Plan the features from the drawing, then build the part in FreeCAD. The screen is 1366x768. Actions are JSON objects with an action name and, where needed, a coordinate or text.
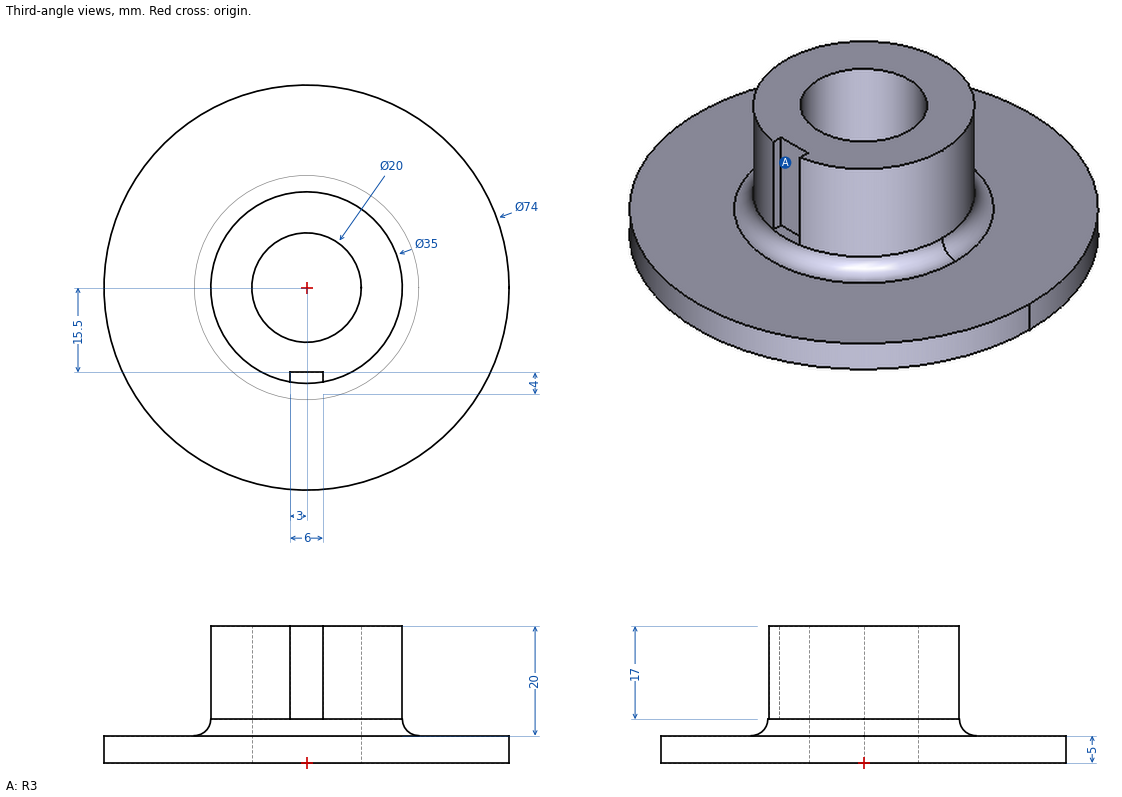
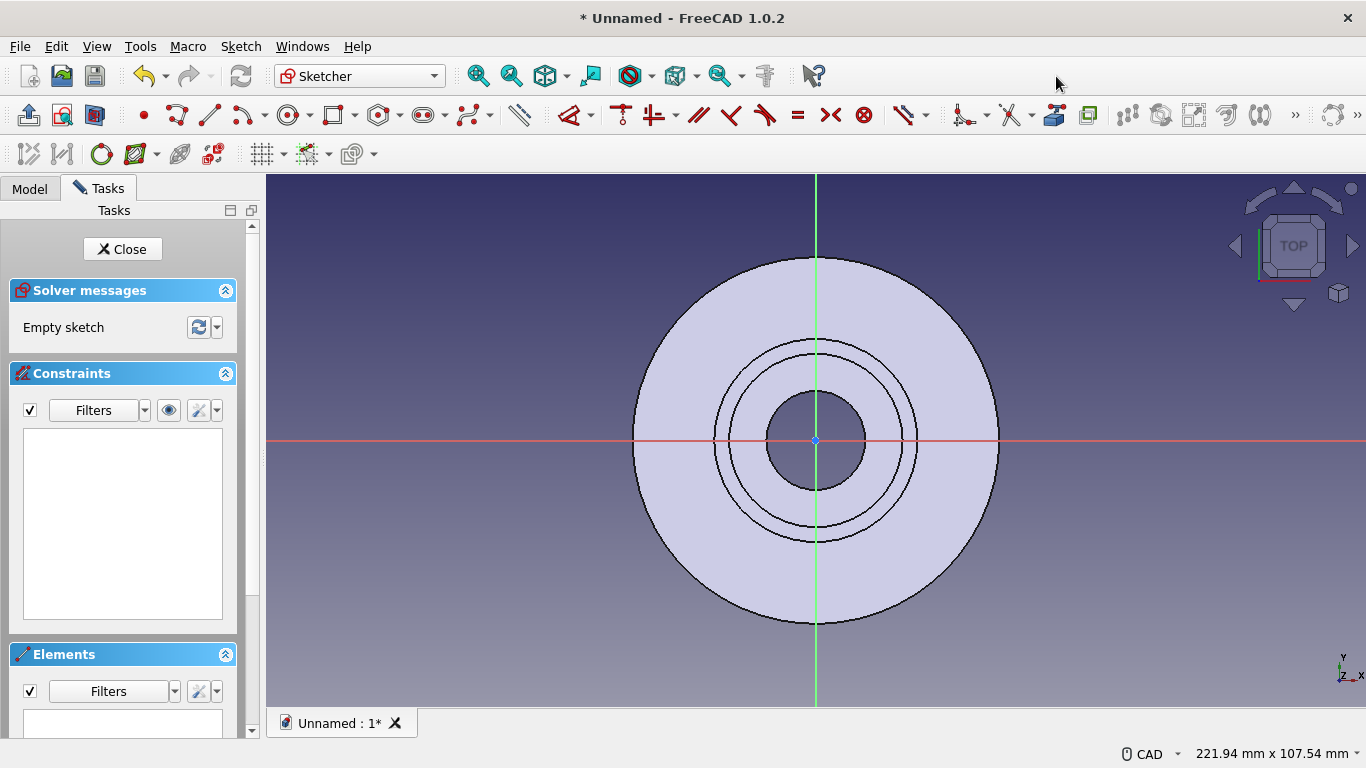
{"action": "scroll", "coordinate": [820, 533], "scroll_direction": "up", "scroll_amount": 14}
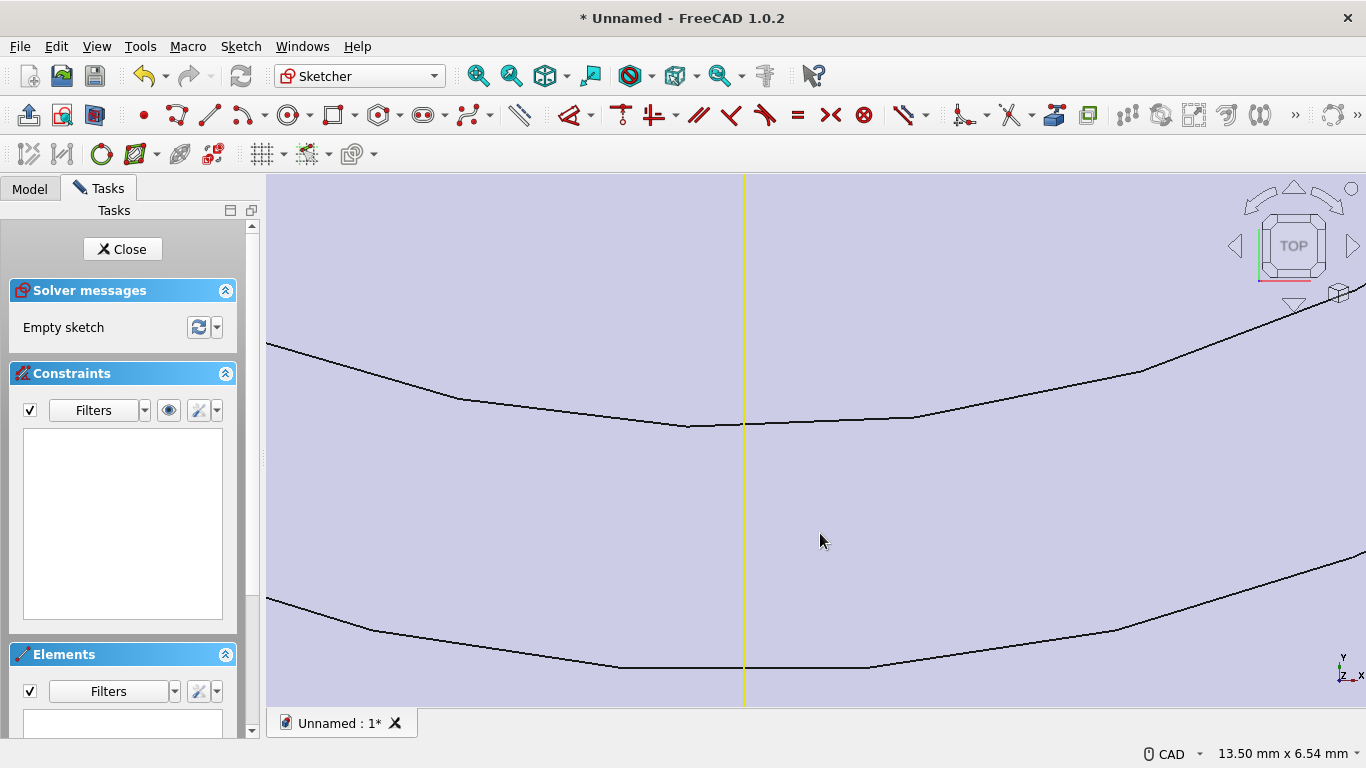
{"action": "left_click", "coordinate": [332, 116]}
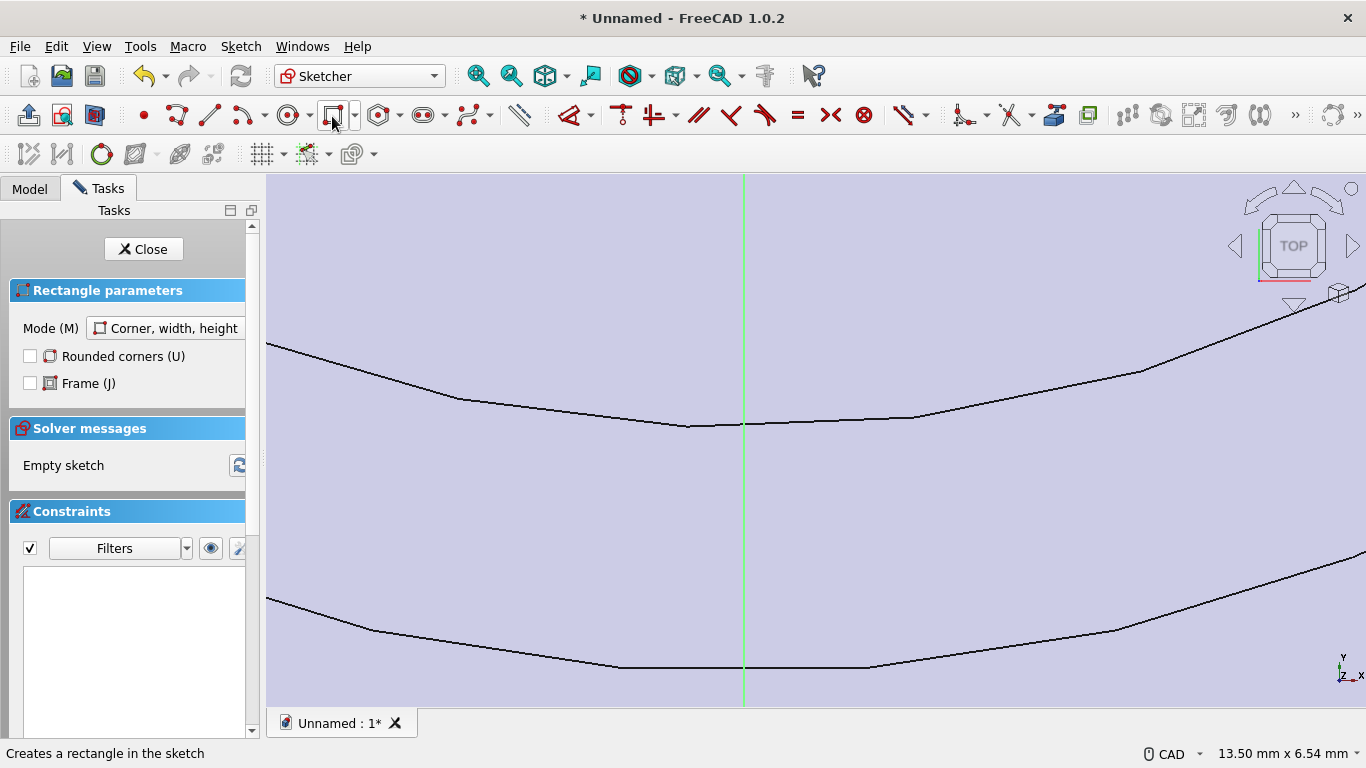
{"action": "left_click", "coordinate": [500, 265]}
{"action": "mouse_move", "coordinate": [989, 591]}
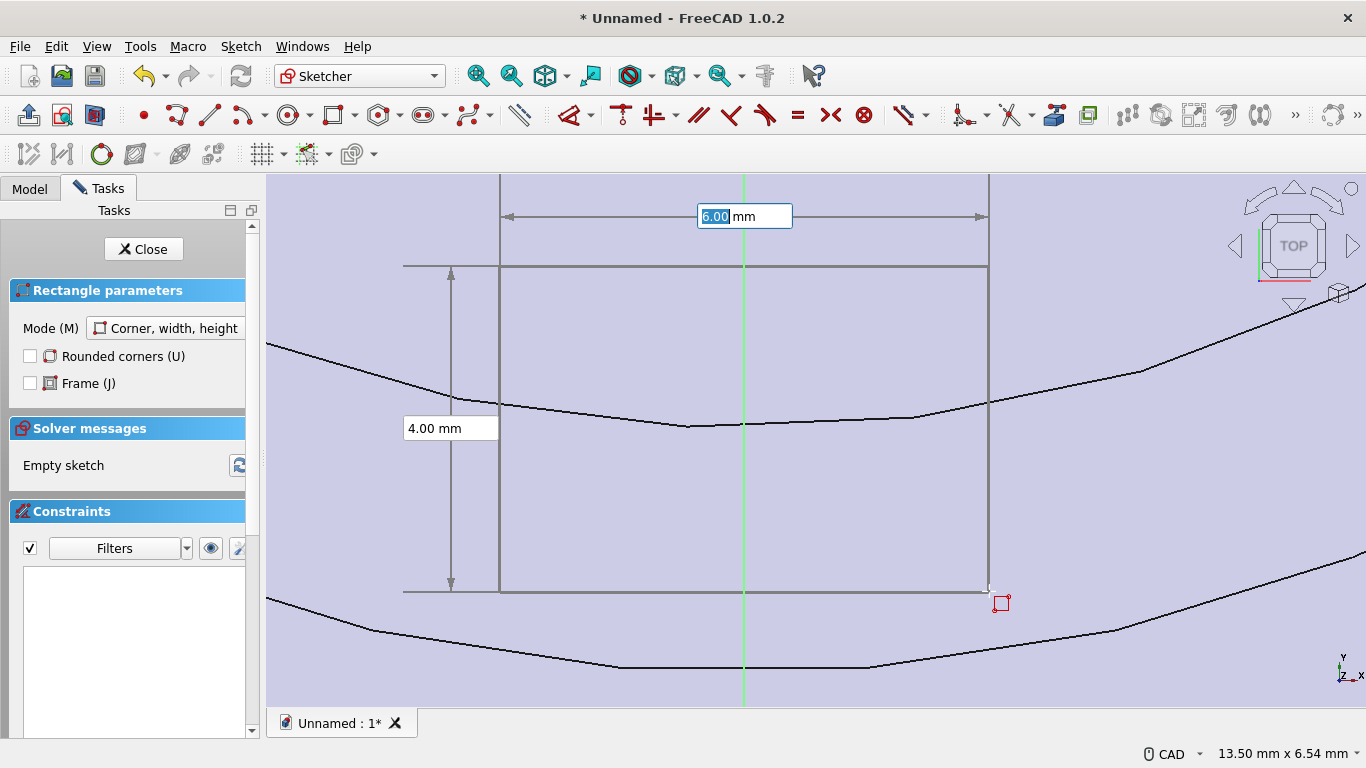
{"action": "type", "text": "6"}
{"action": "key", "text": "Tab"}
{"action": "type", "text": "4"}
{"action": "key", "text": "Return"}
{"action": "key", "text": "Escape"}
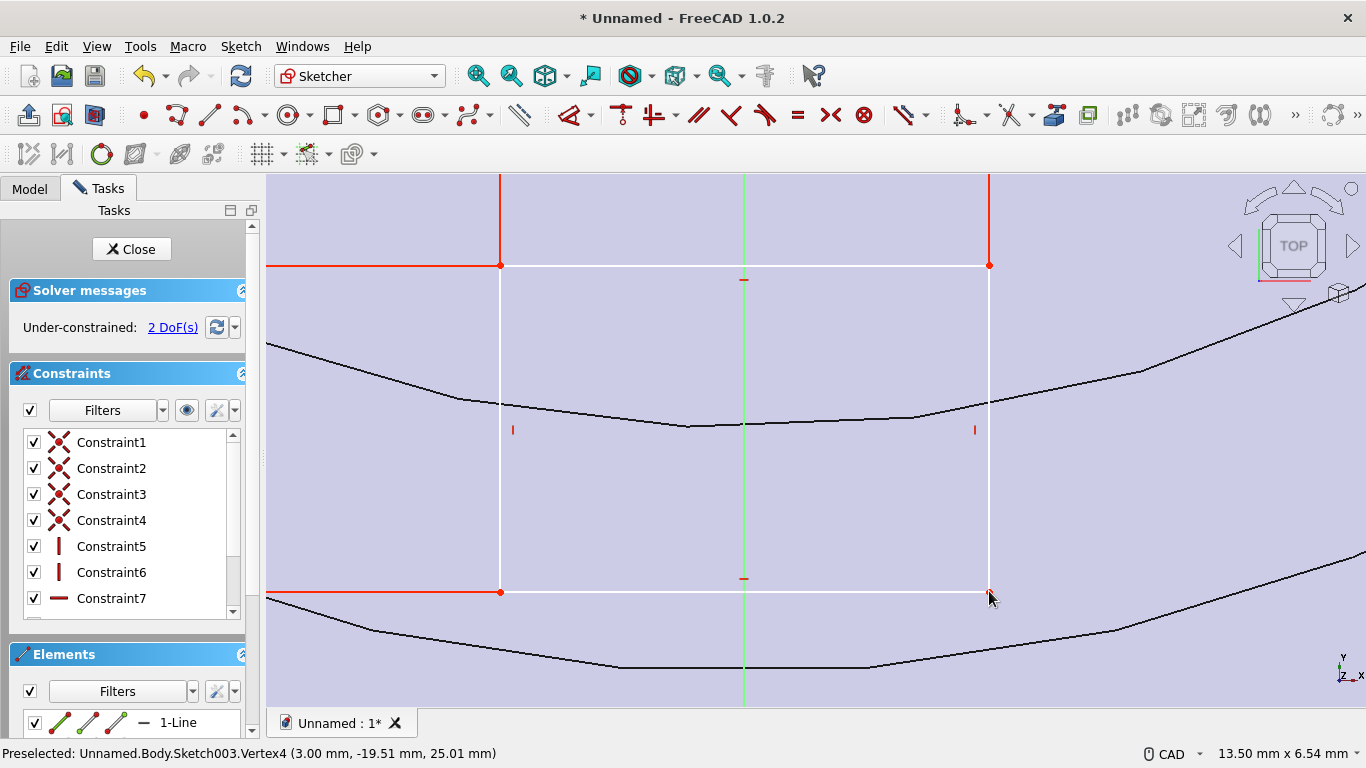
{"action": "left_click", "coordinate": [568, 116]}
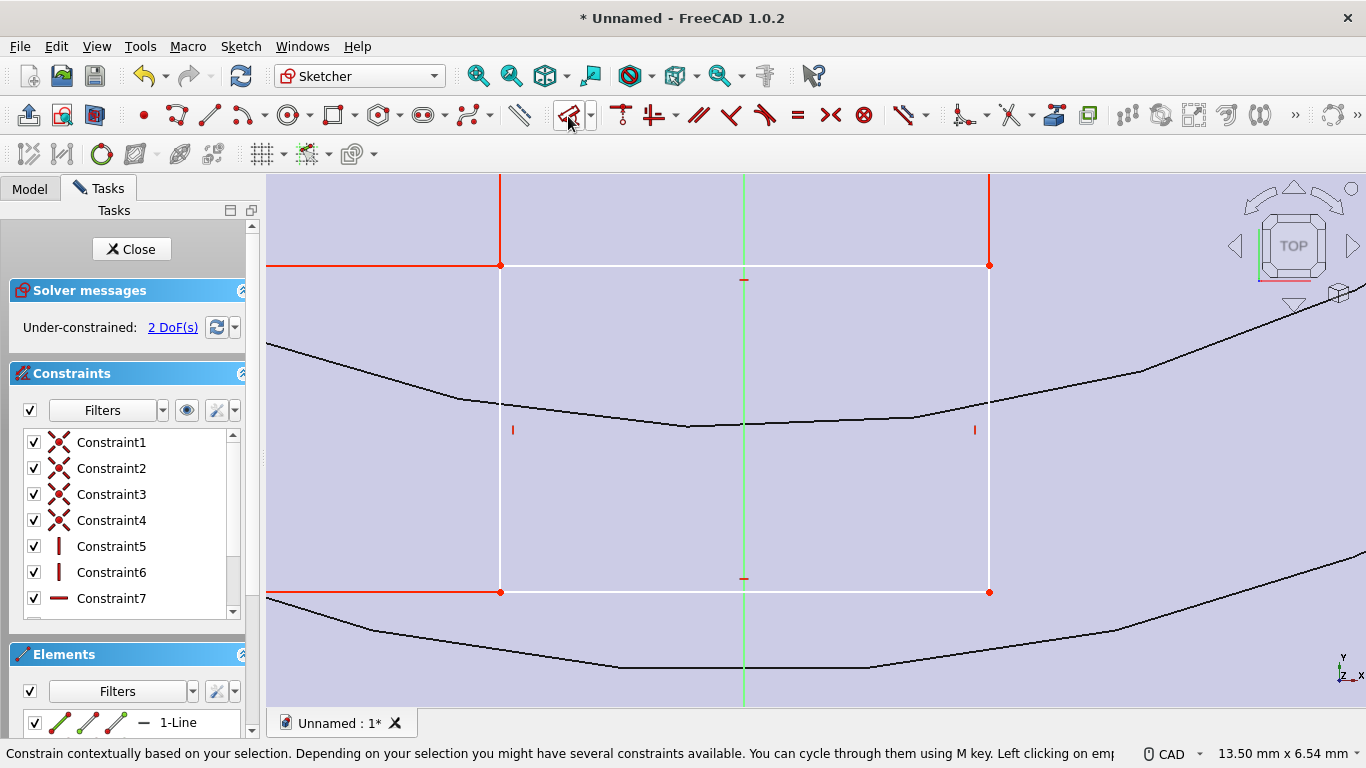
{"action": "left_click", "coordinate": [500, 266]}
{"action": "left_click", "coordinate": [622, 300]}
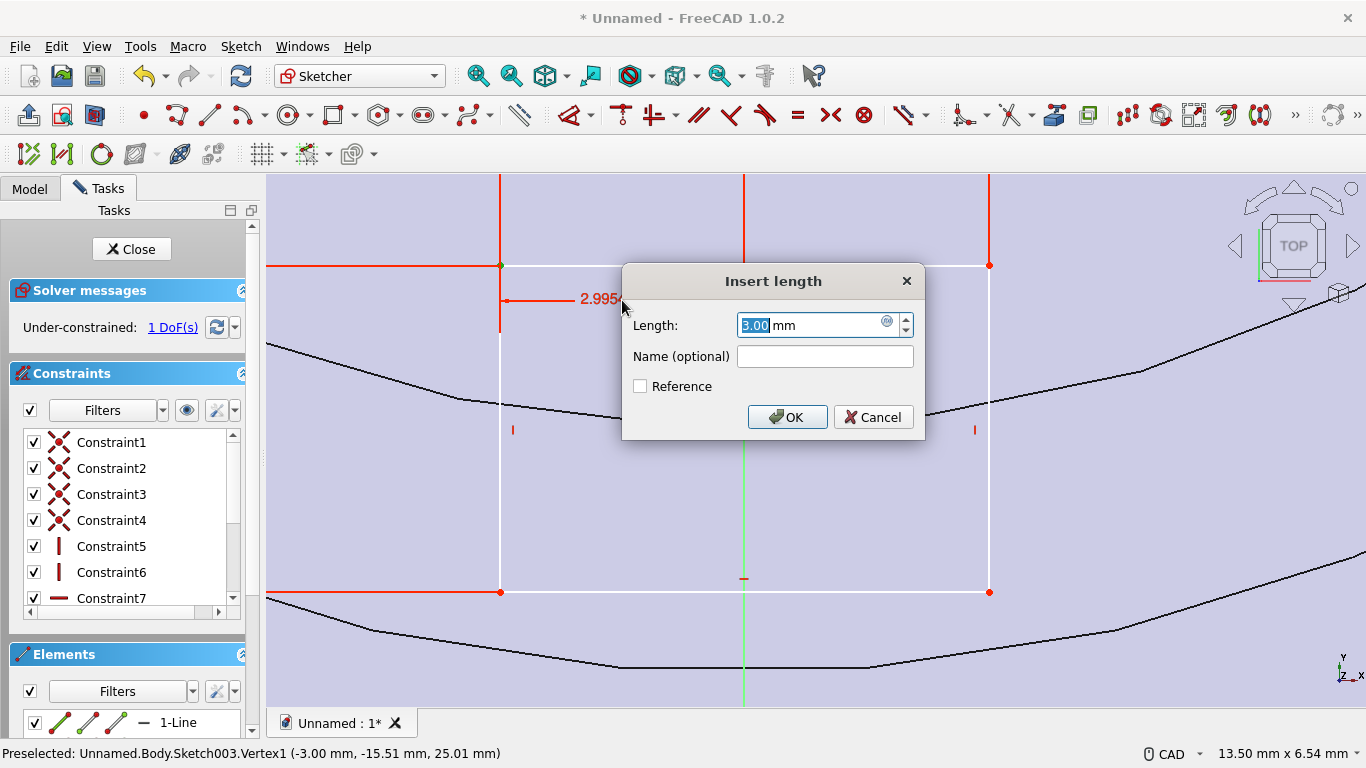
{"action": "type", "text": "3"}
{"action": "key", "text": "Return"}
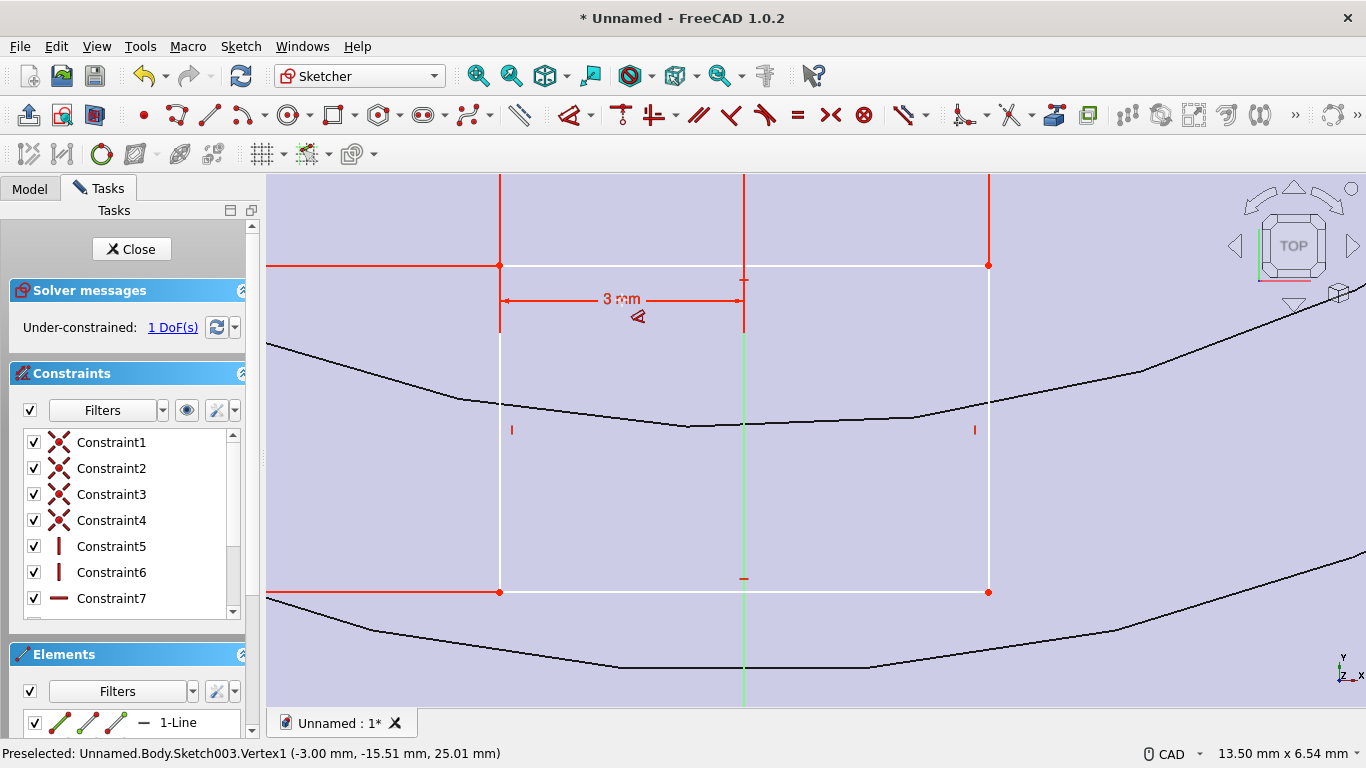
{"action": "left_click", "coordinate": [500, 266]}
{"action": "left_click", "coordinate": [466, 234]}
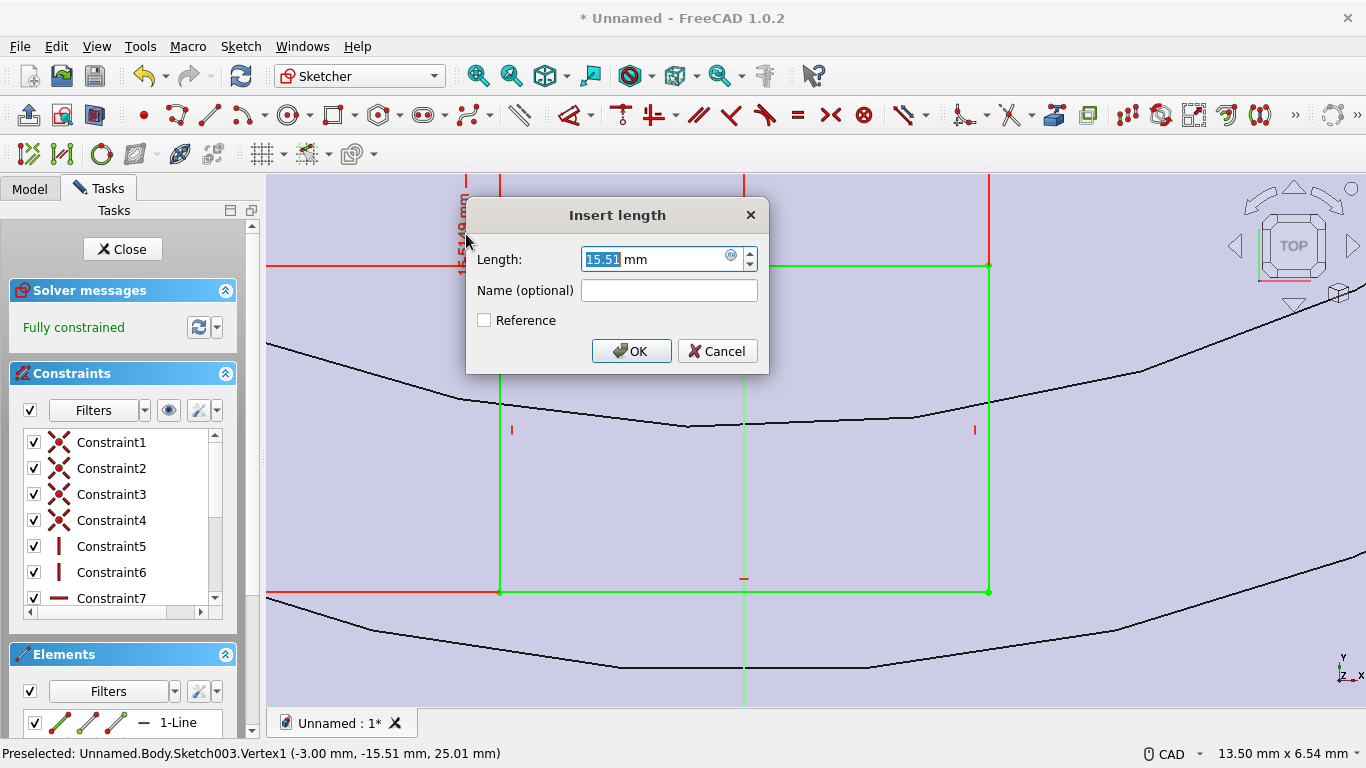
{"action": "type", "text": "15.5"}
{"action": "key", "text": "Return"}
{"action": "key", "text": "Escape"}